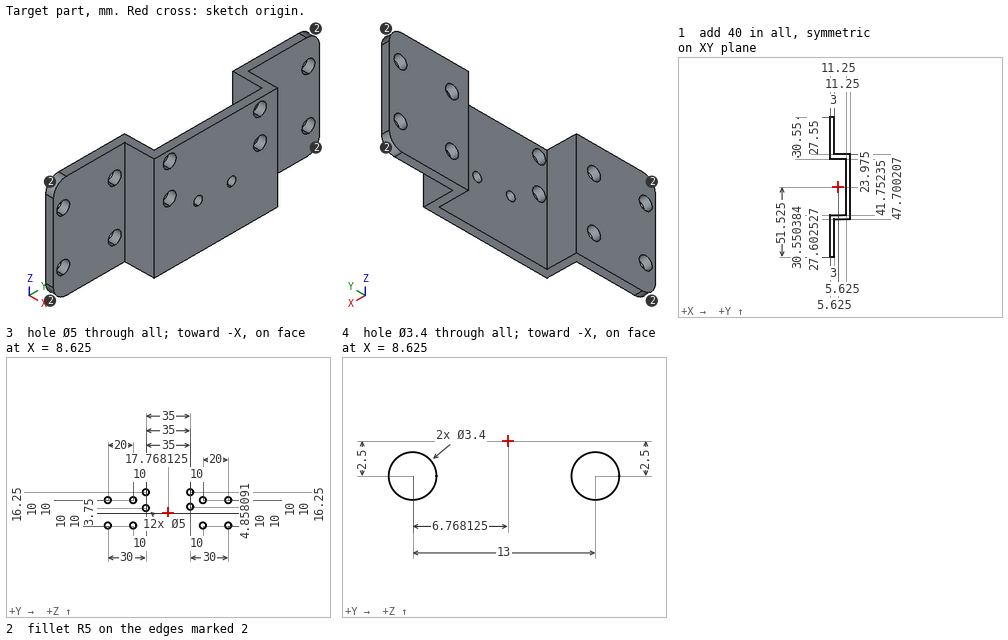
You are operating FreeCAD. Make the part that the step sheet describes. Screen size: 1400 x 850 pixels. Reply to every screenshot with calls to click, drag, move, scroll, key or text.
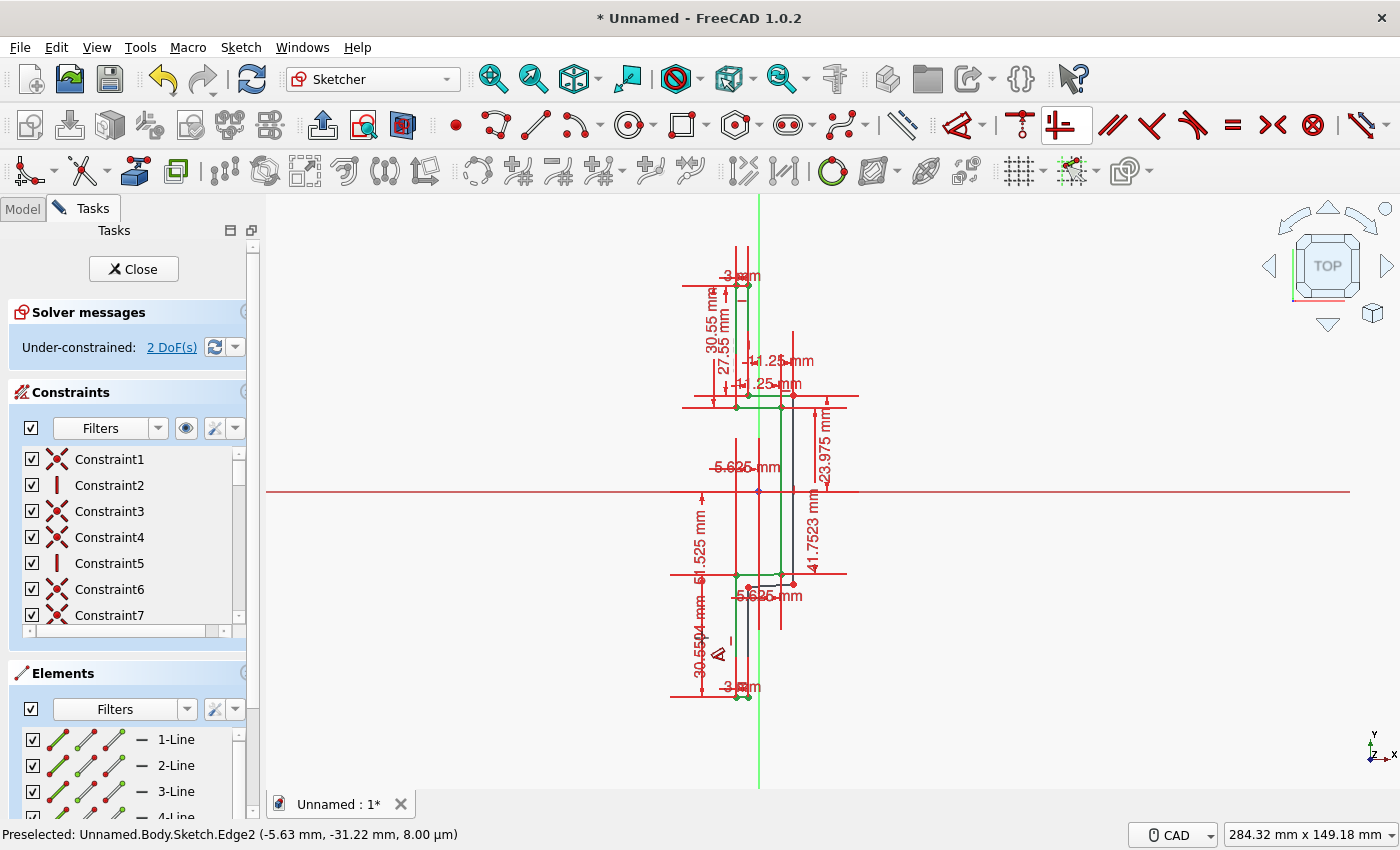
scroll(748, 664, up, 2)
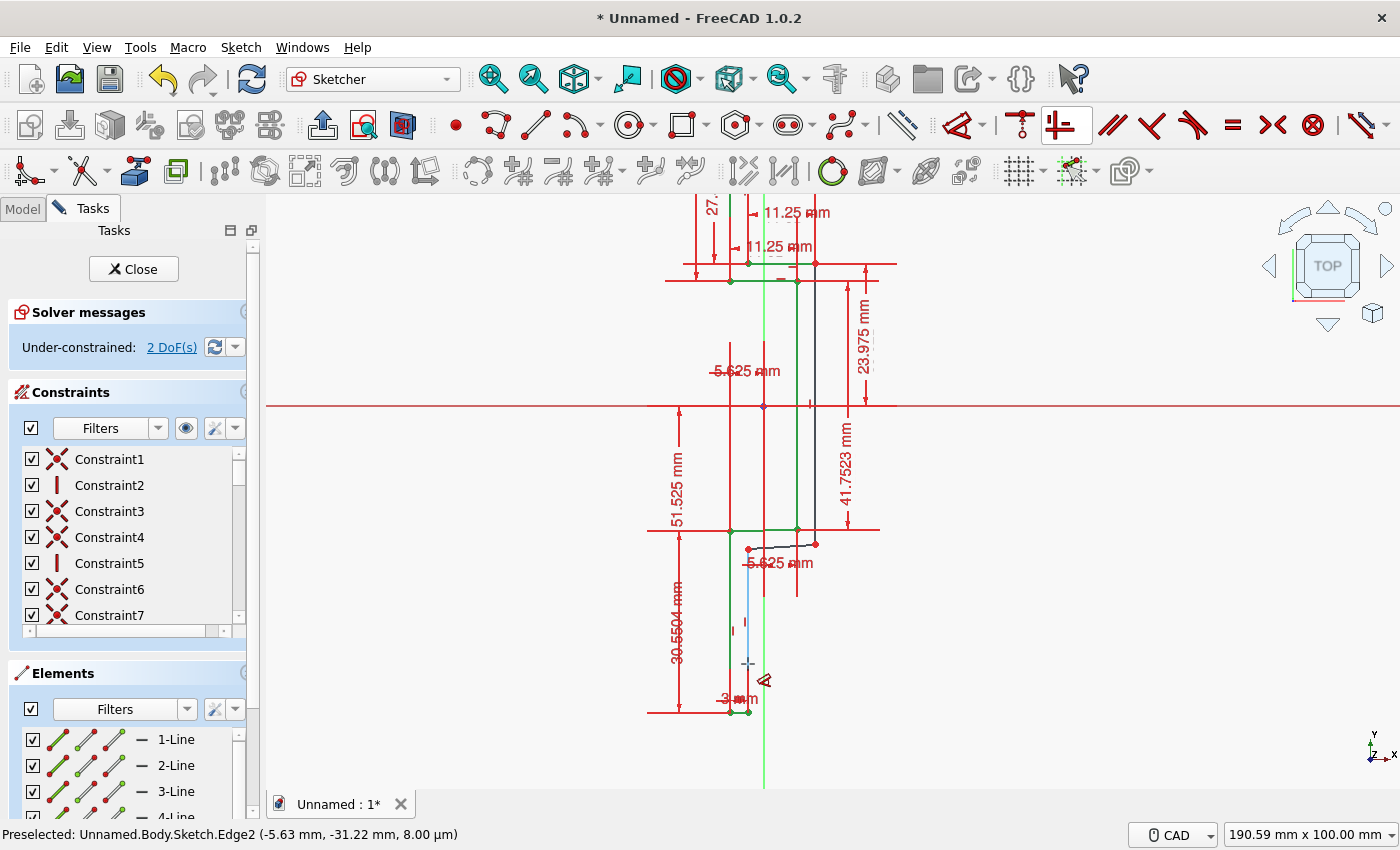
click(748, 664)
click(714, 593)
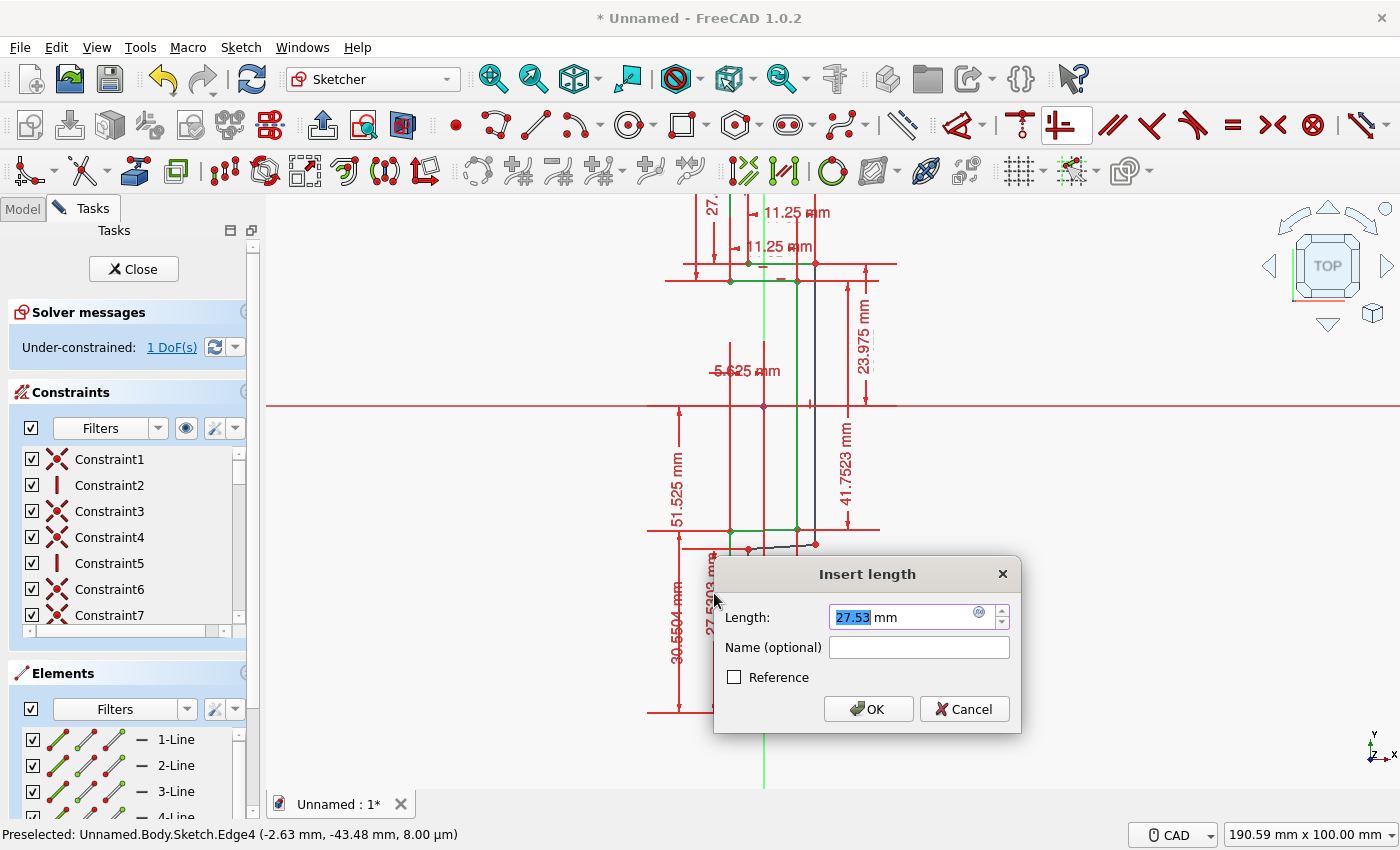
text(27.602527)
key(Return)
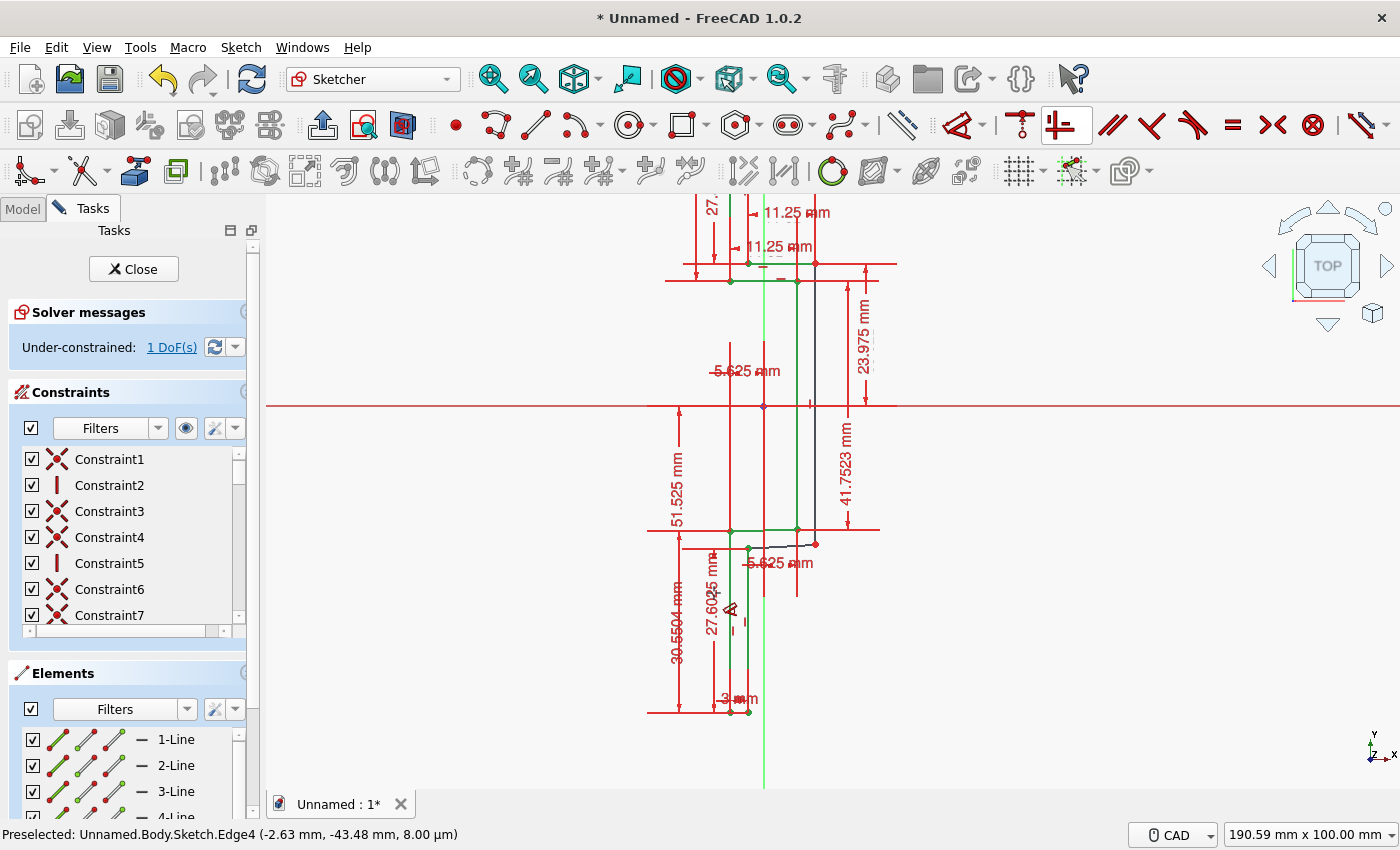
click(815, 461)
click(849, 306)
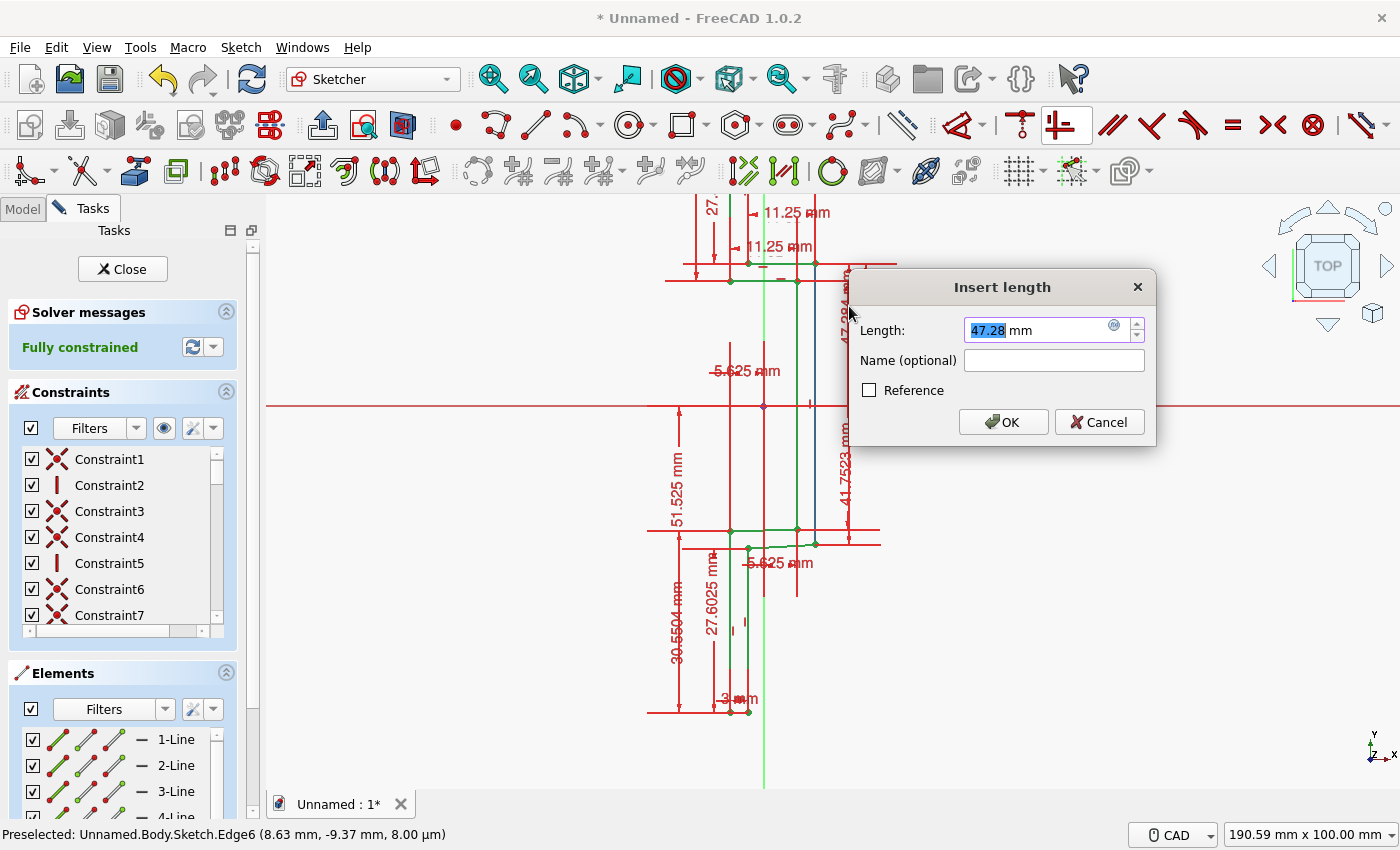
text(47.700207)
key(Return)
key(Escape)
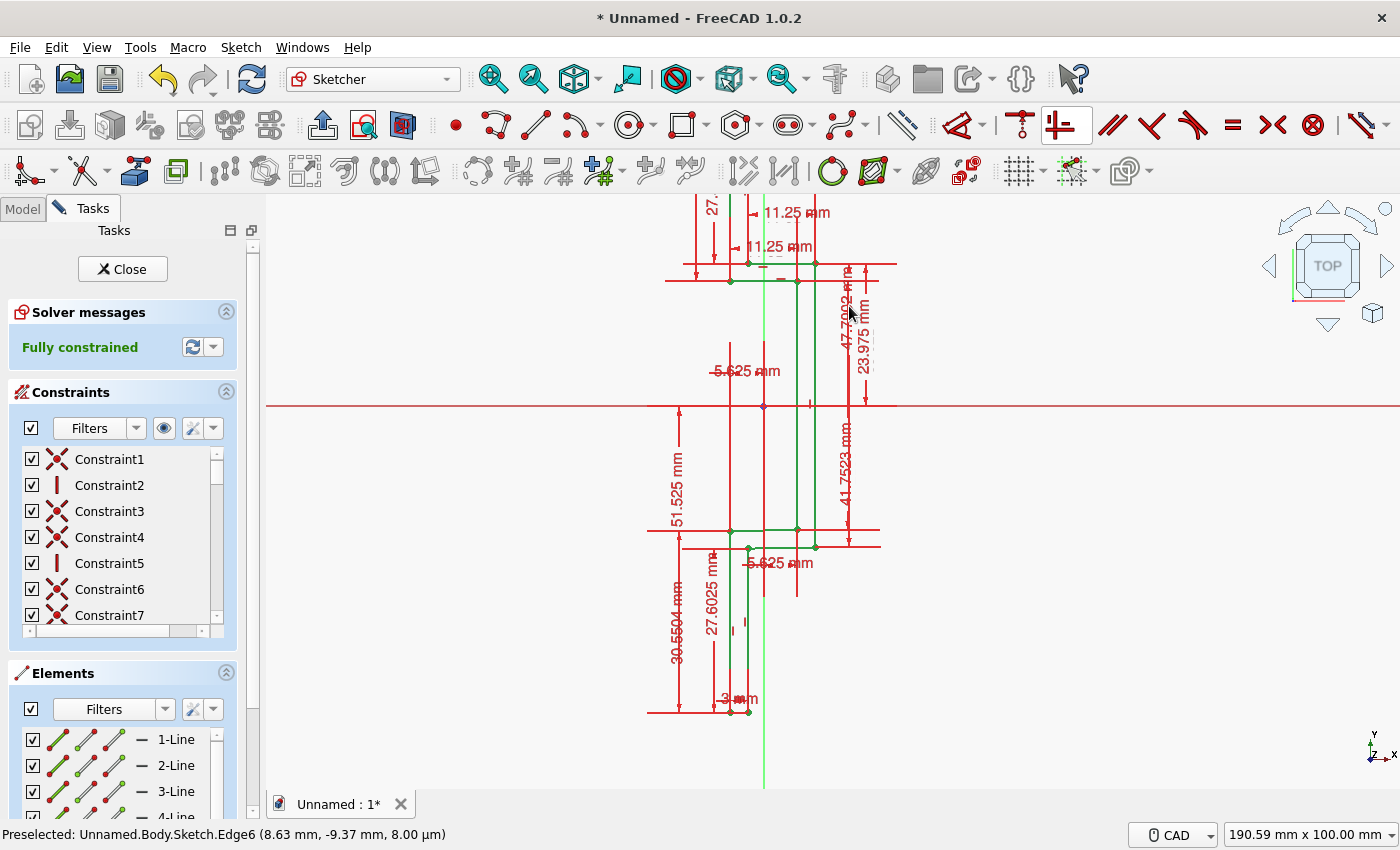
click(123, 269)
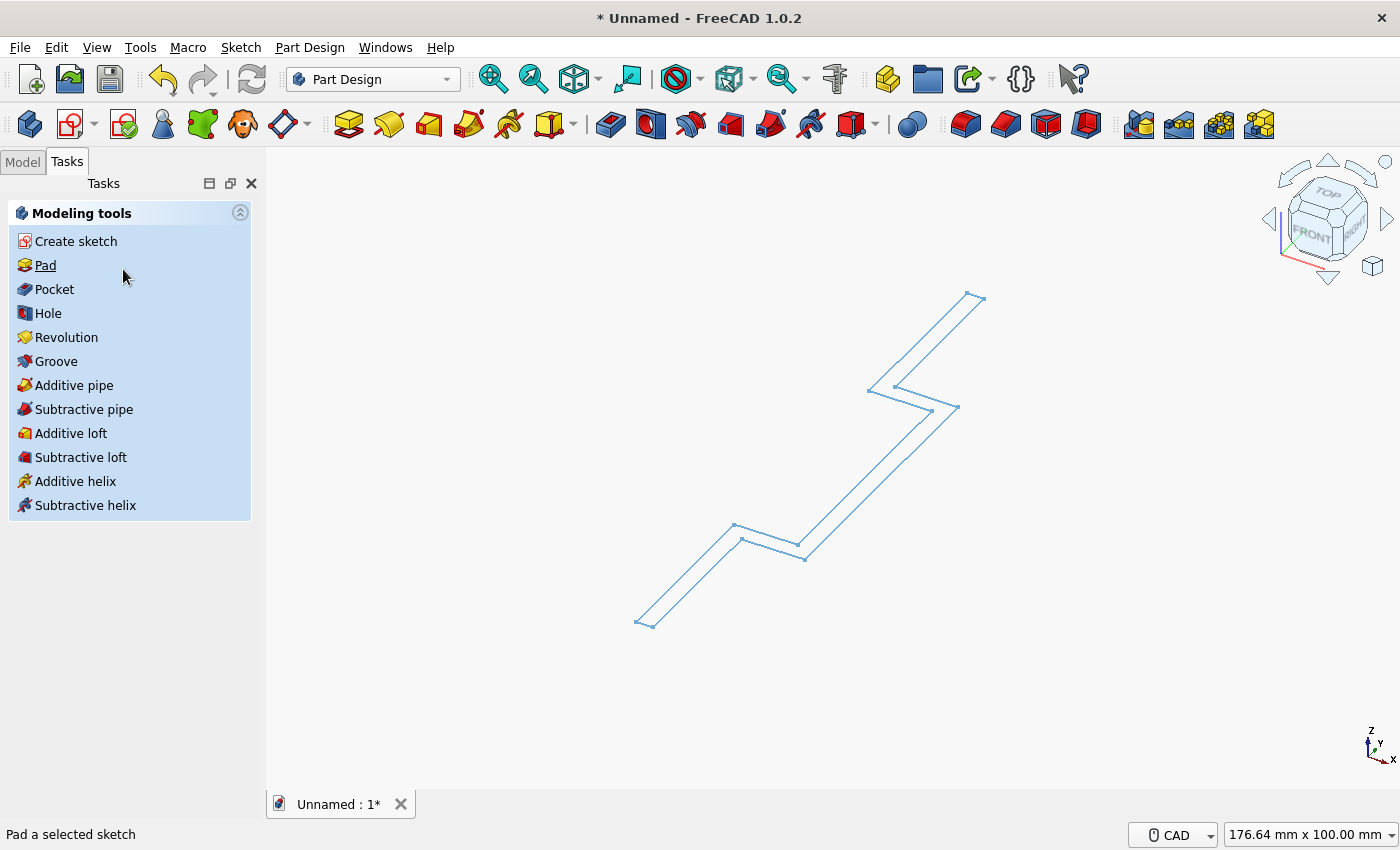
click(350, 124)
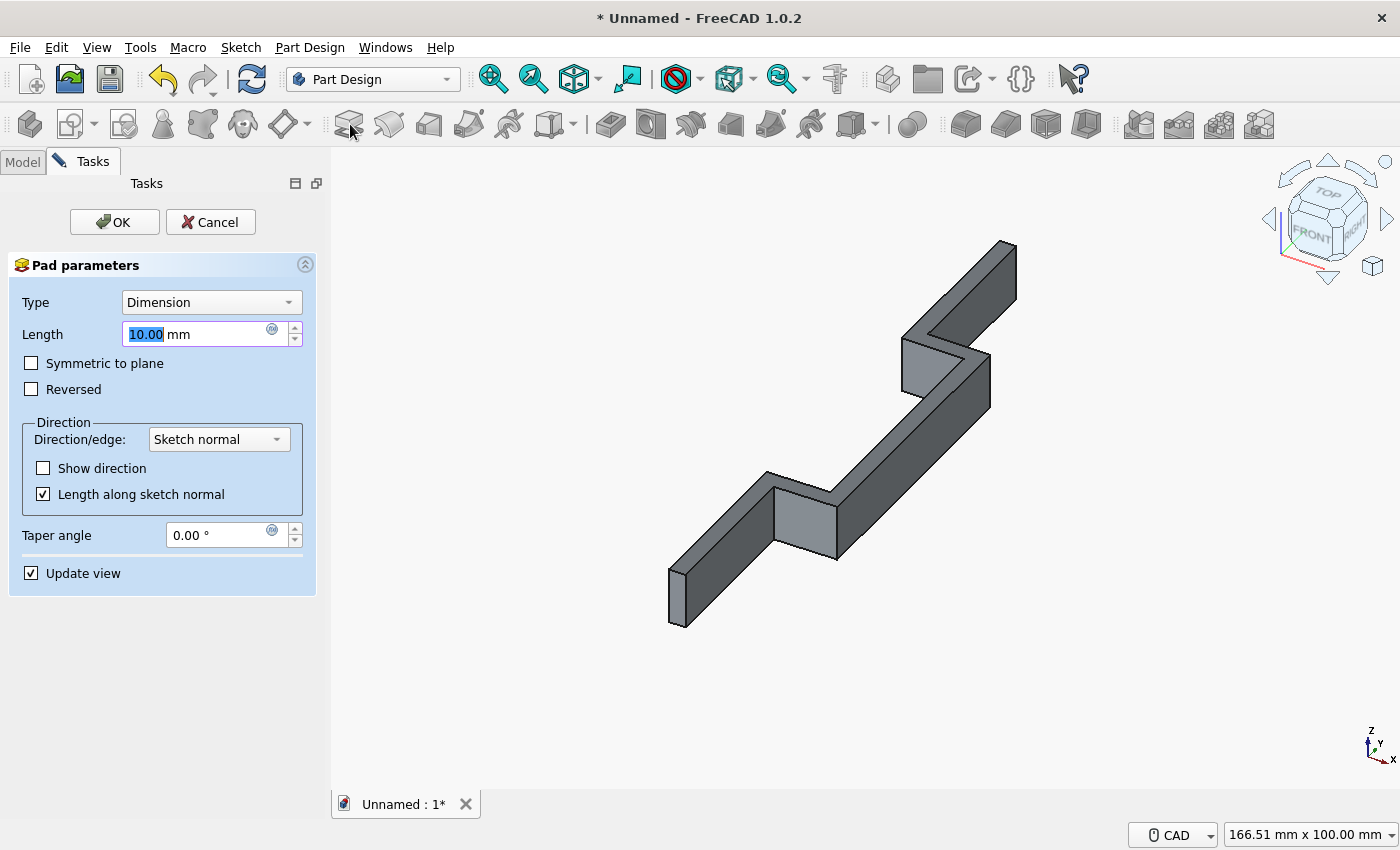
text(40)
key(Tab)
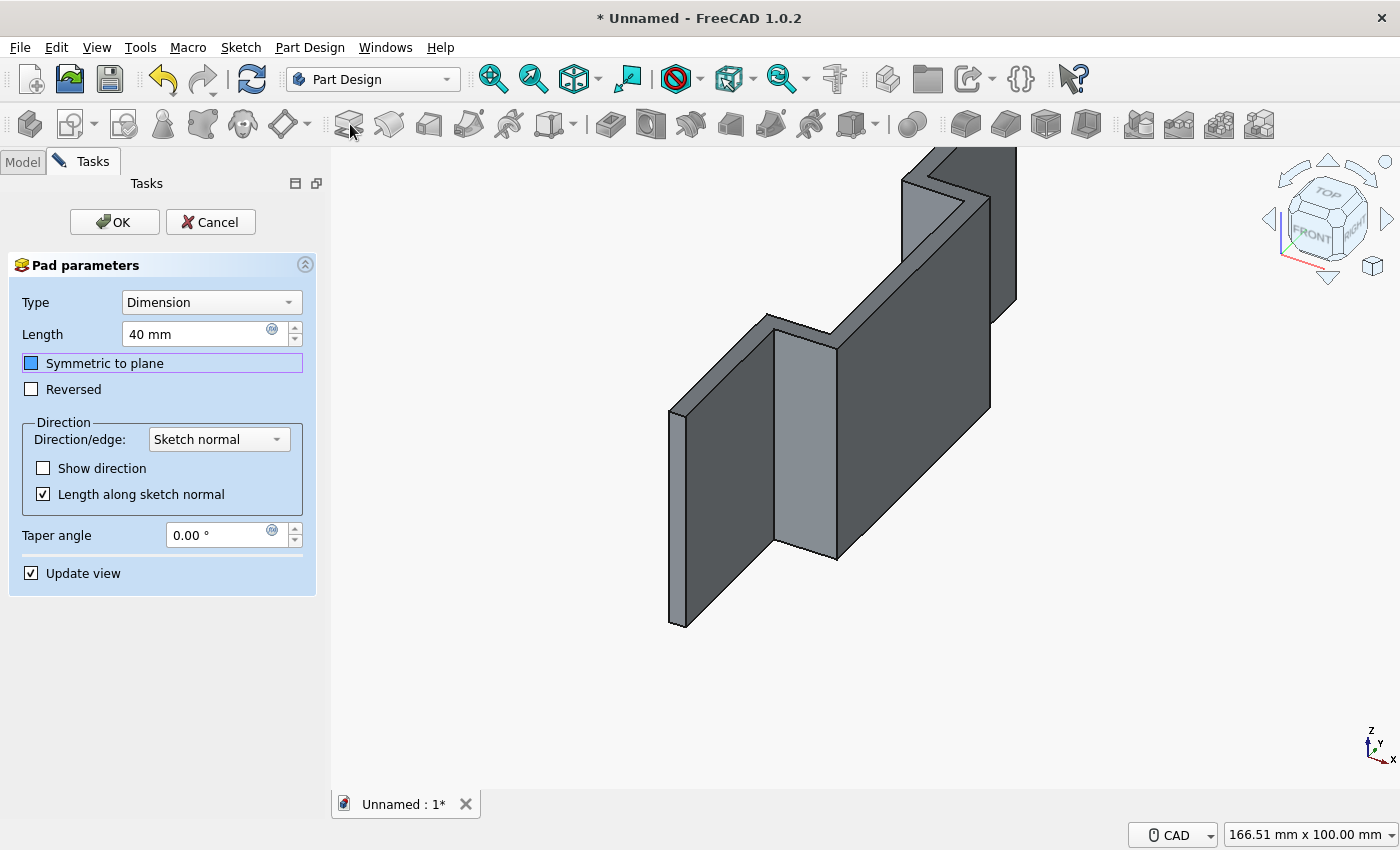
click(30, 363)